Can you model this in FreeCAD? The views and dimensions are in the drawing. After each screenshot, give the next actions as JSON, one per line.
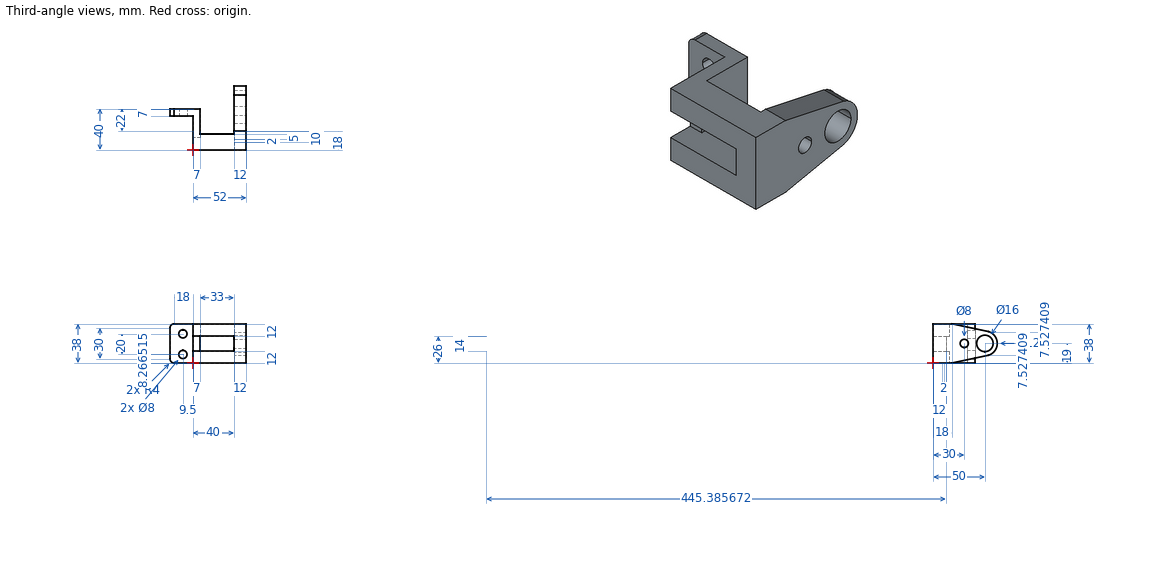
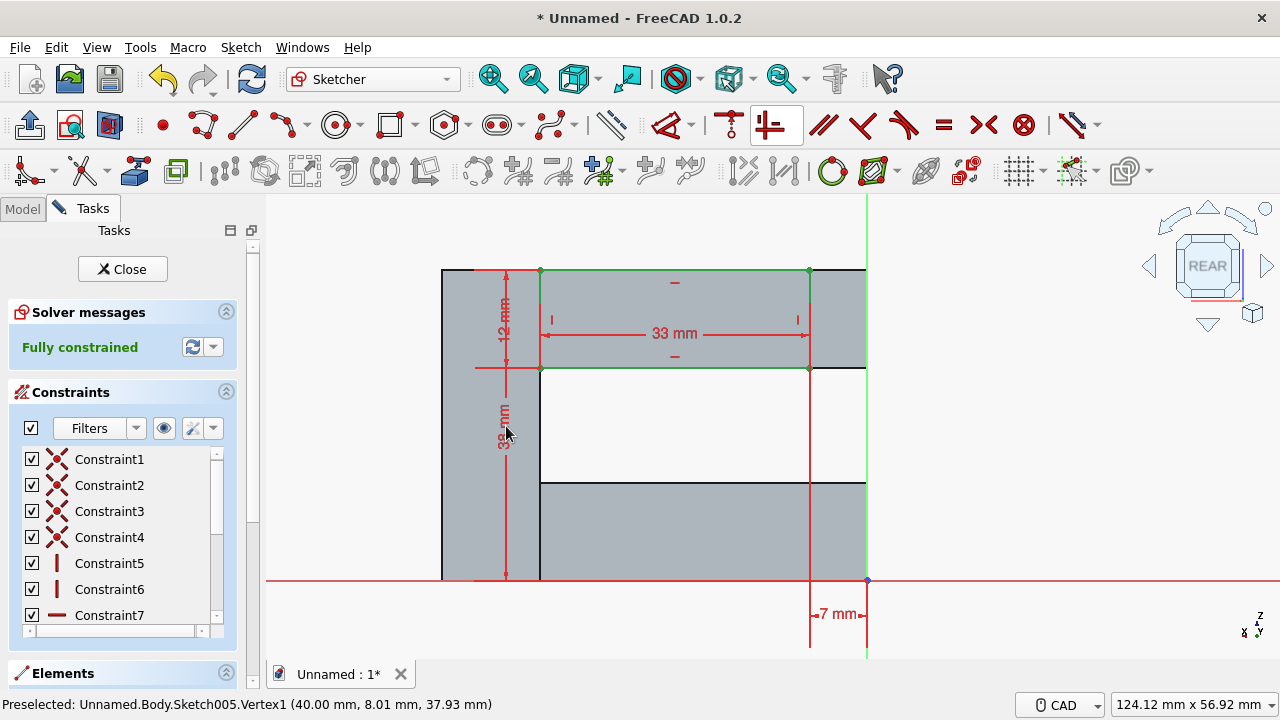
{"action": "left_click", "coordinate": [123, 269]}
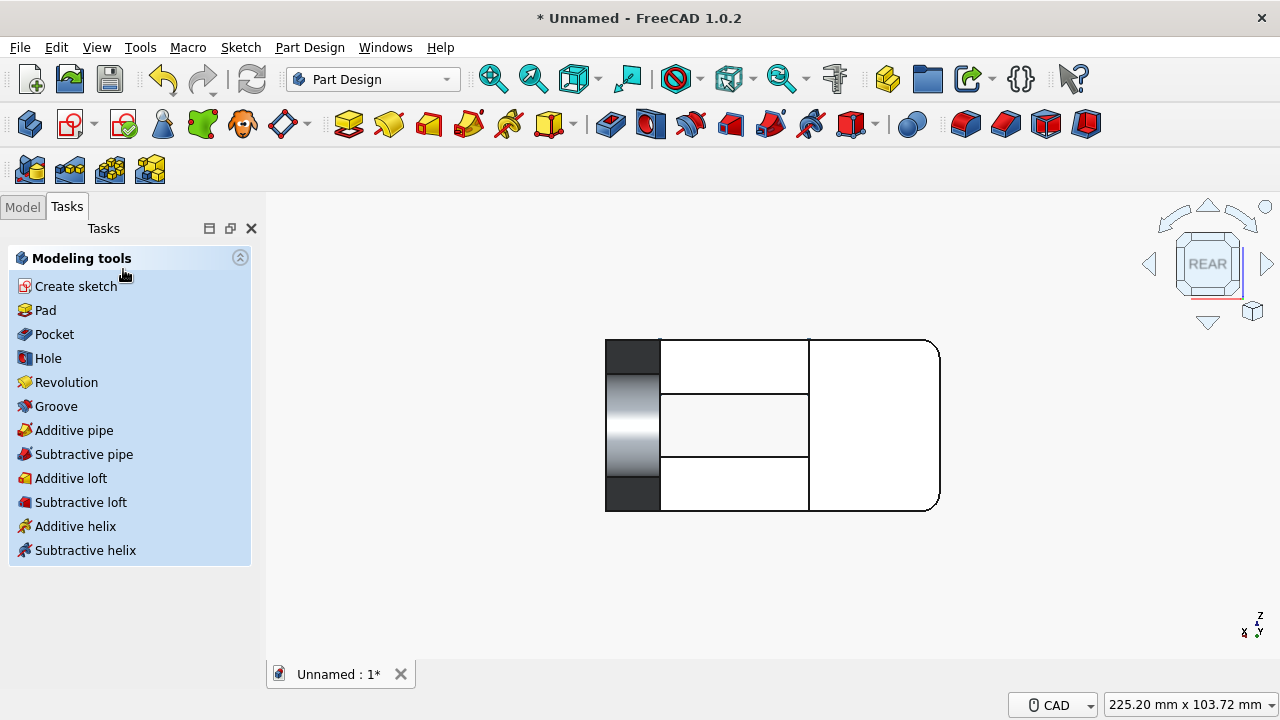
{"action": "left_click", "coordinate": [350, 124]}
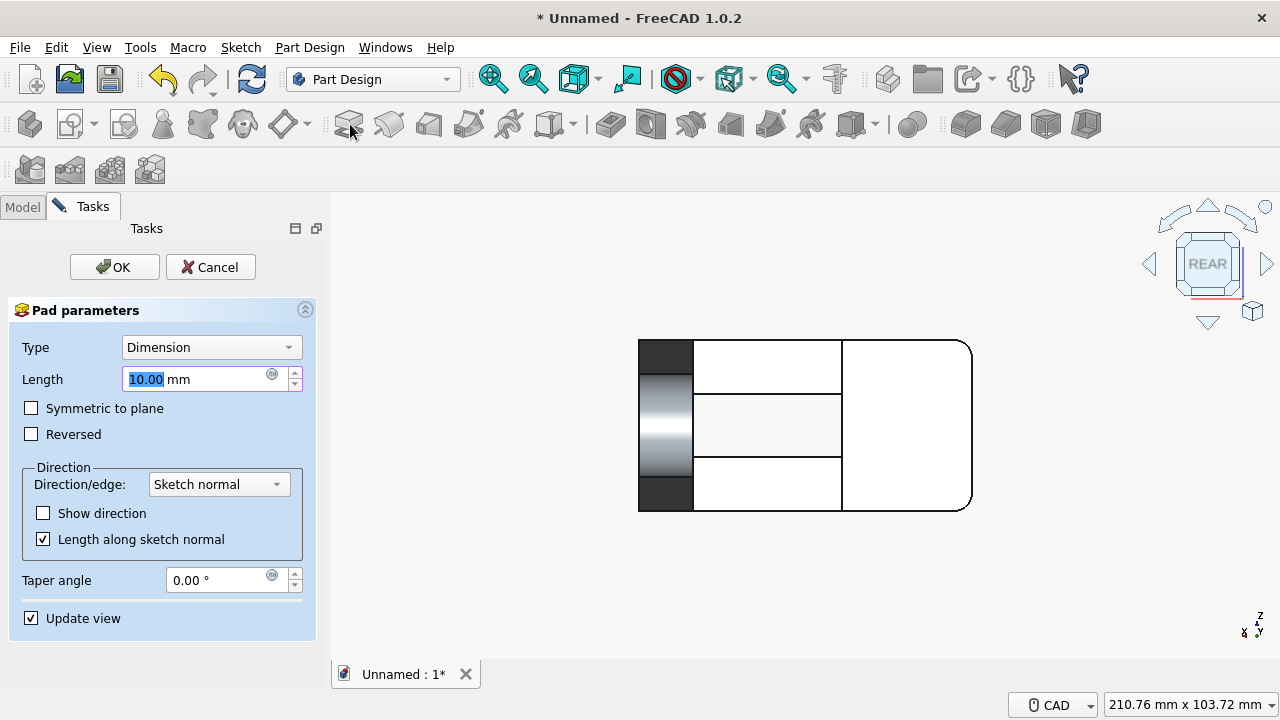
{"action": "type", "text": "2"}
{"action": "key", "text": "Tab"}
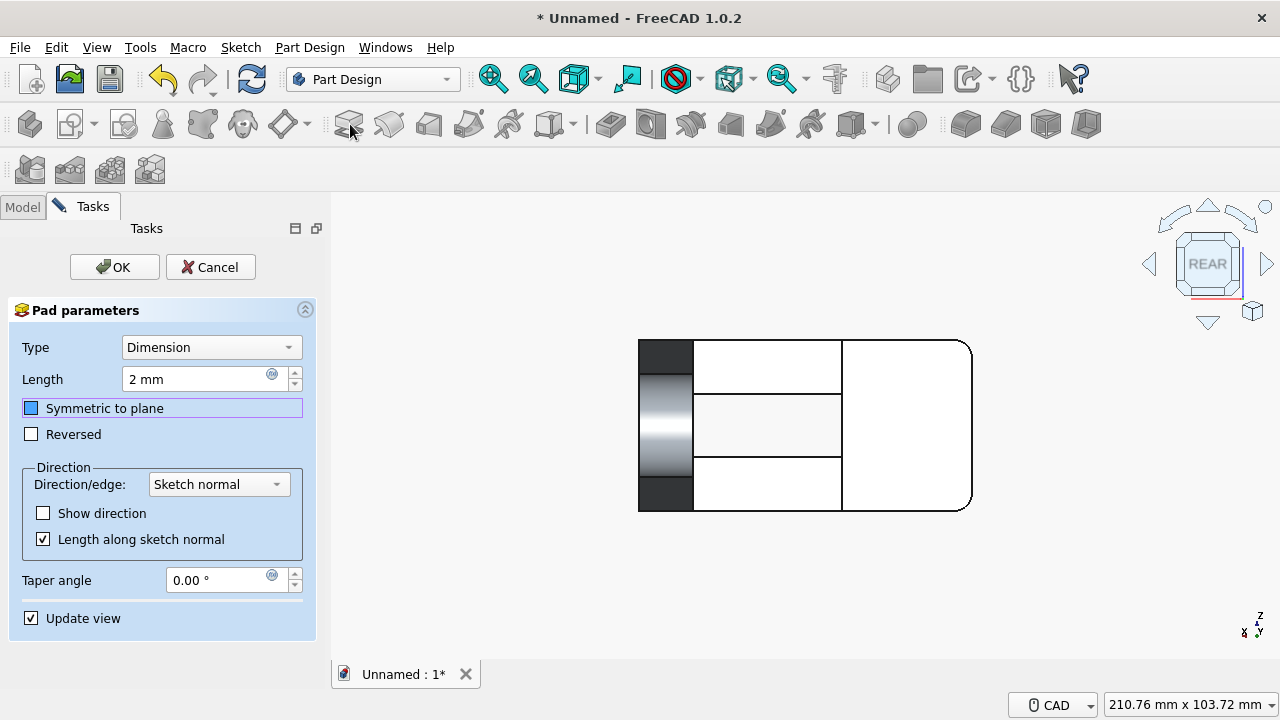
{"action": "left_click", "coordinate": [115, 267]}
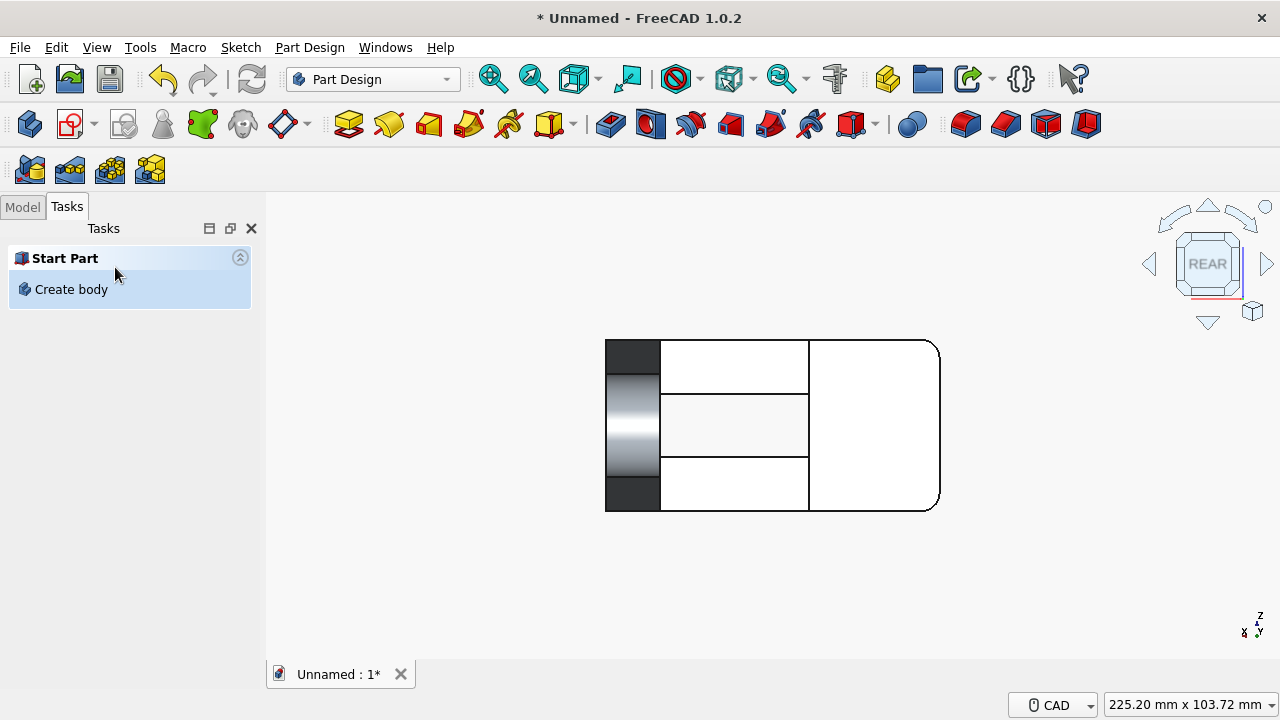
{"action": "left_click", "coordinate": [494, 80]}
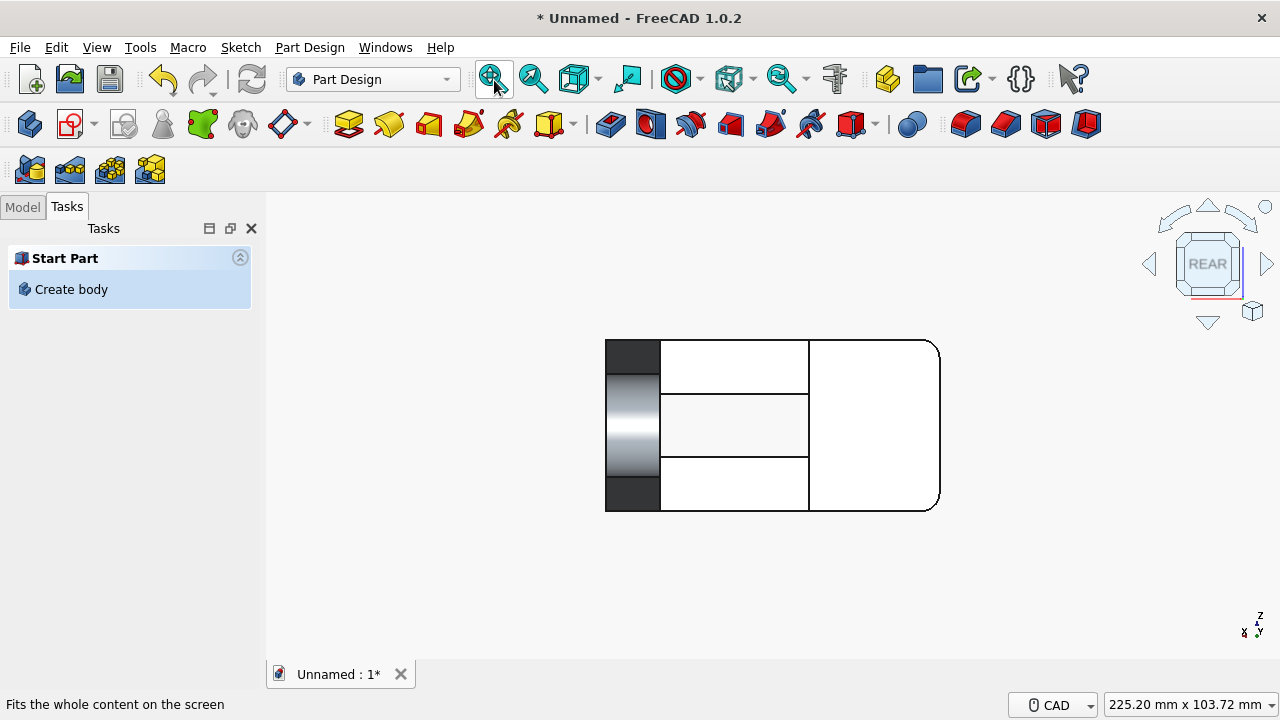
{"action": "left_click", "coordinate": [692, 483]}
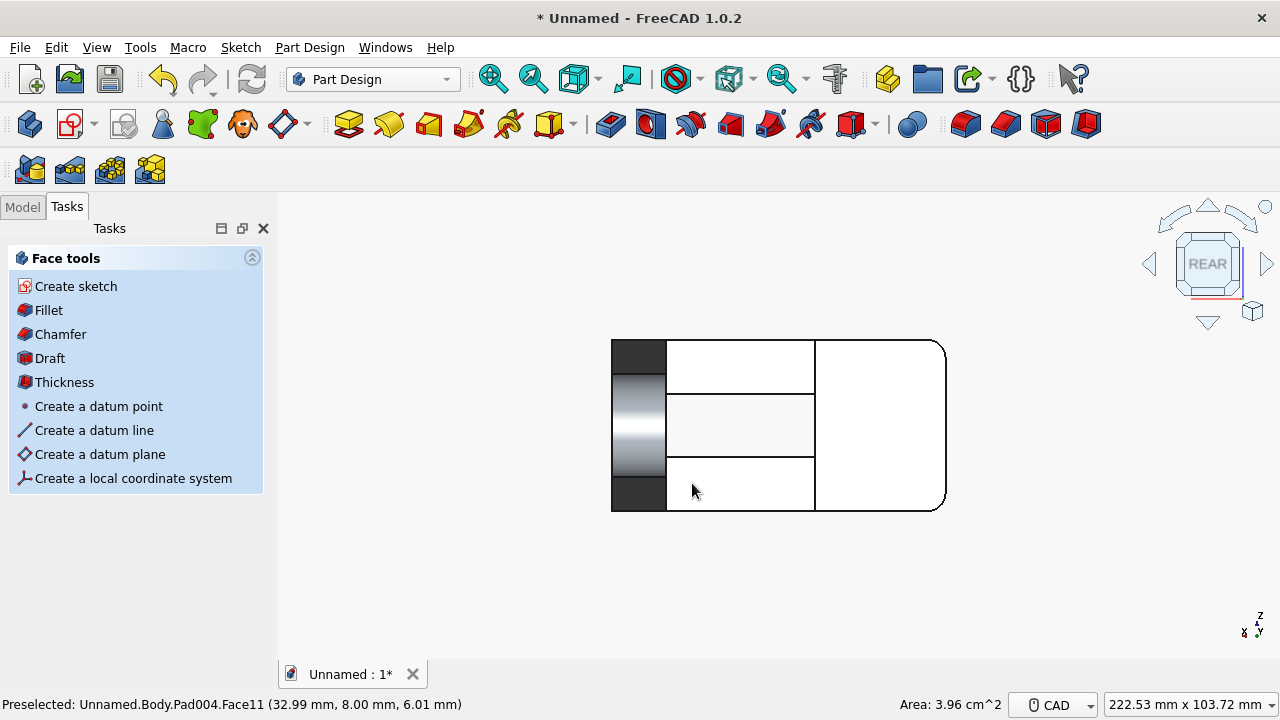
{"action": "left_click", "coordinate": [70, 124]}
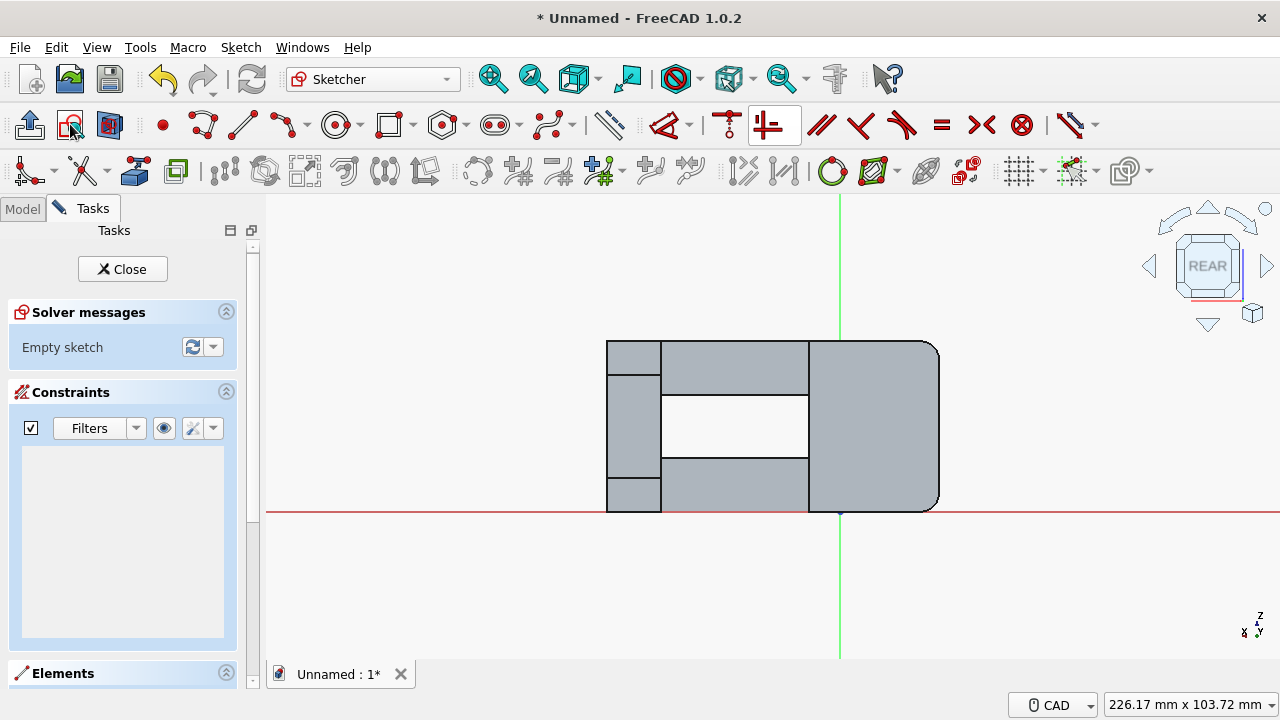
{"action": "left_click", "coordinate": [110, 126]}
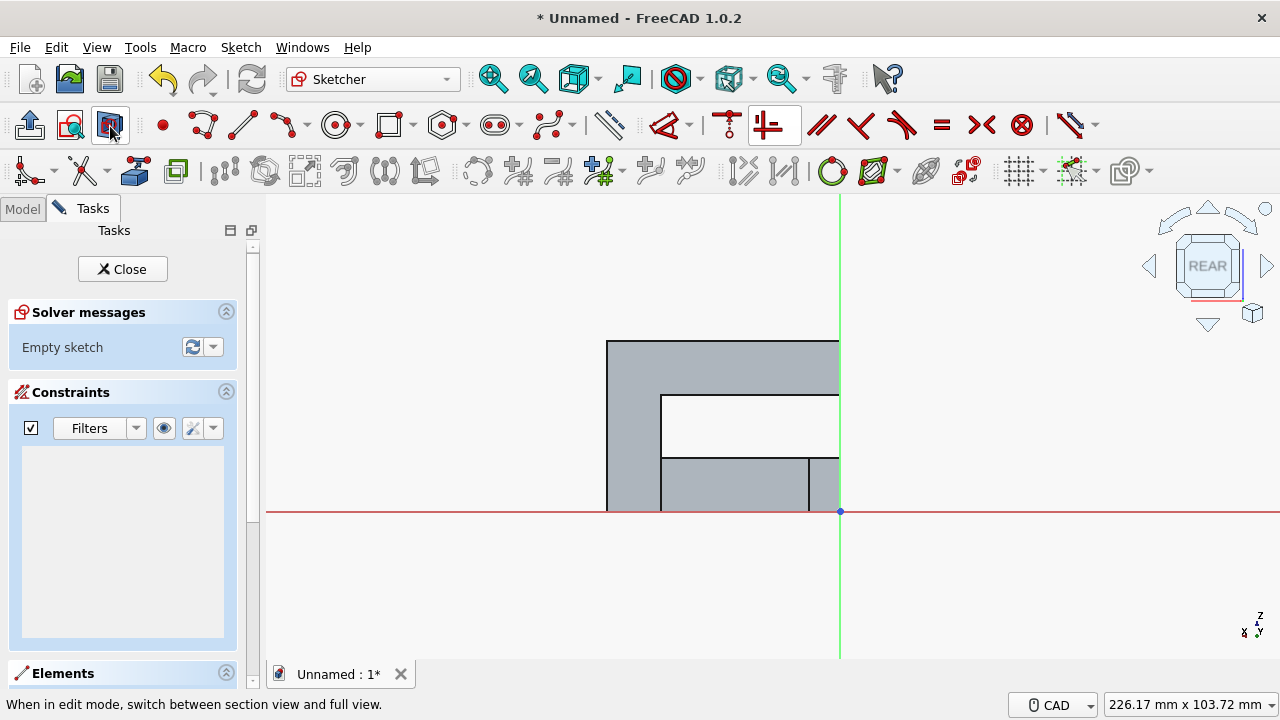
{"action": "scroll", "coordinate": [770, 510], "scroll_direction": "up", "scroll_amount": 6}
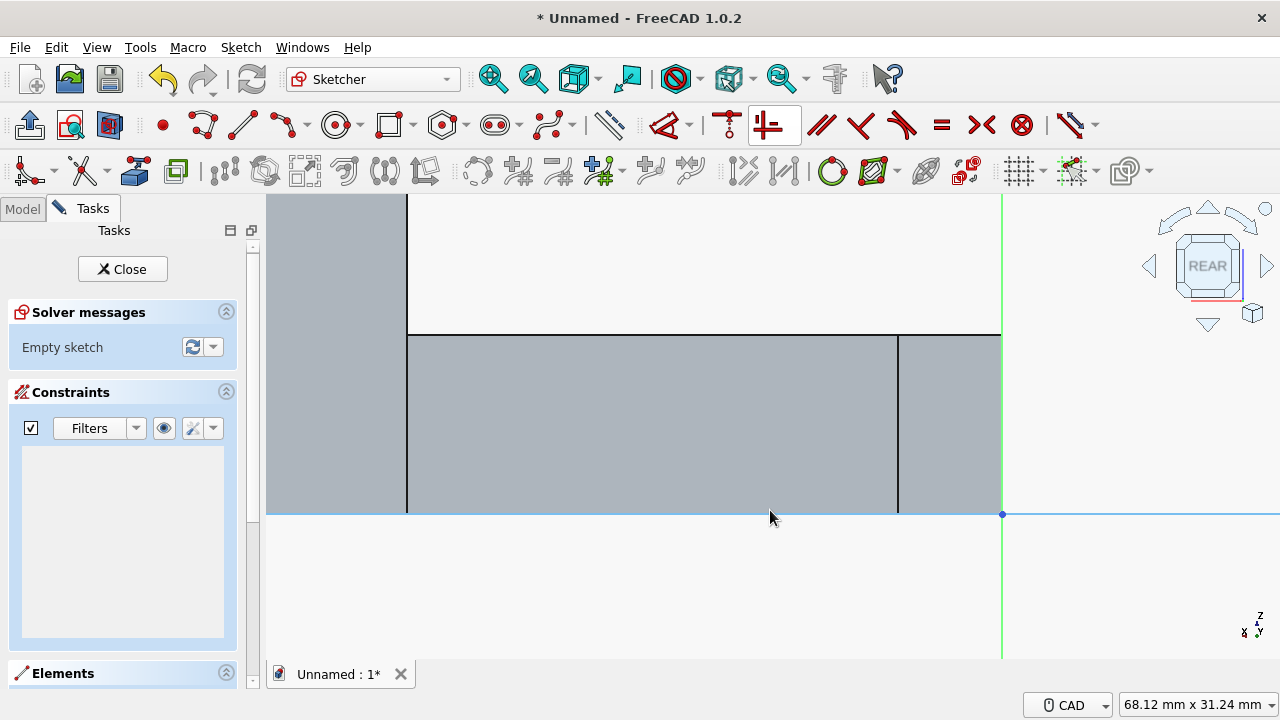
{"action": "left_click", "coordinate": [390, 126]}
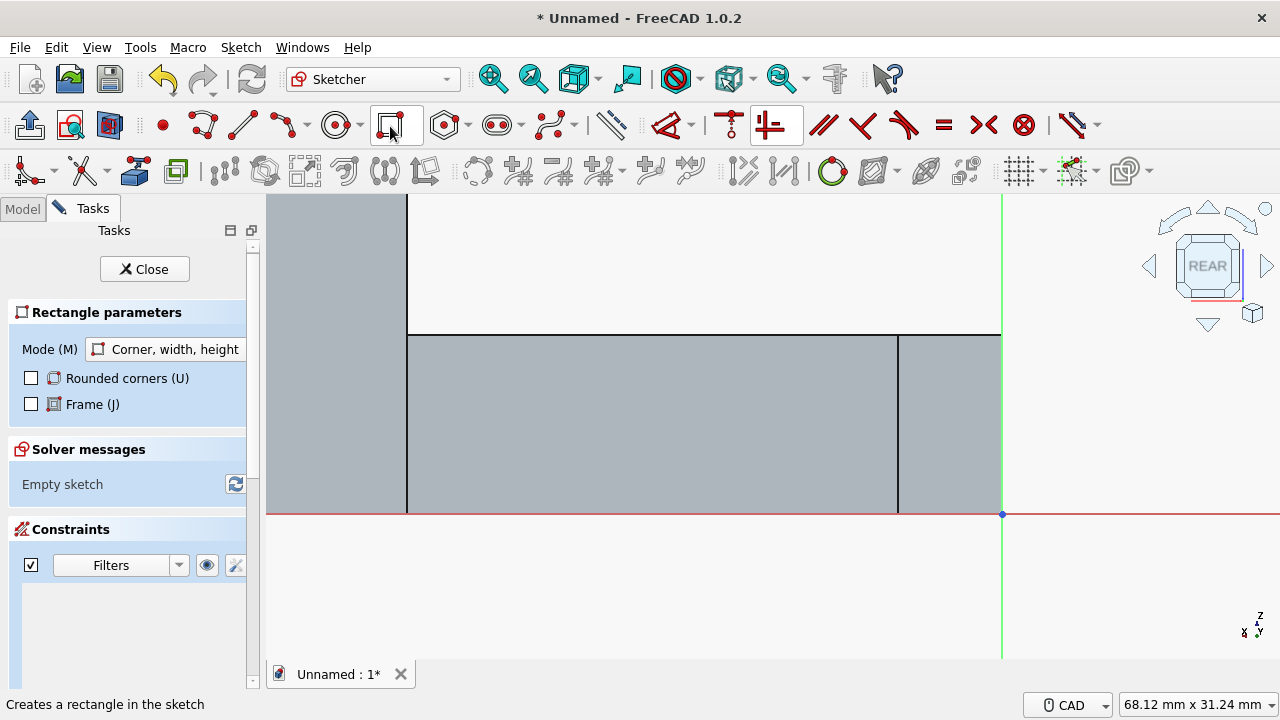
{"action": "left_click", "coordinate": [407, 335]}
{"action": "left_click", "coordinate": [898, 514]}
{"action": "key", "text": "Escape"}